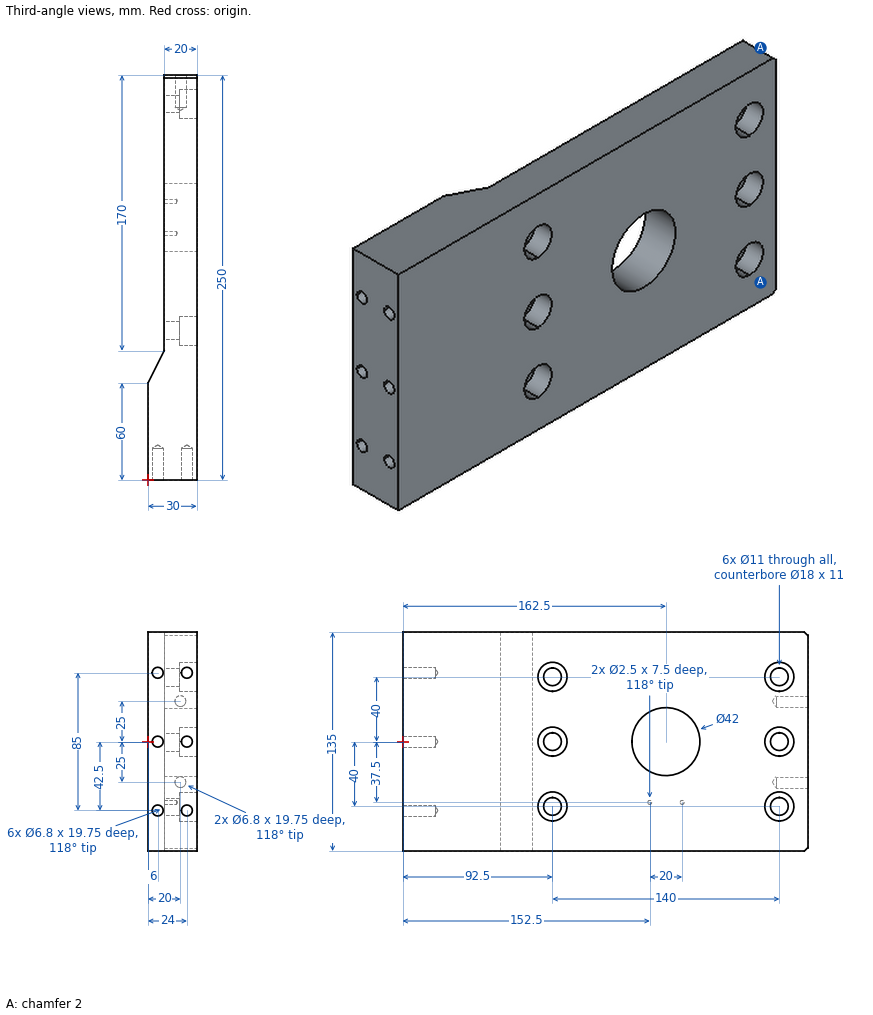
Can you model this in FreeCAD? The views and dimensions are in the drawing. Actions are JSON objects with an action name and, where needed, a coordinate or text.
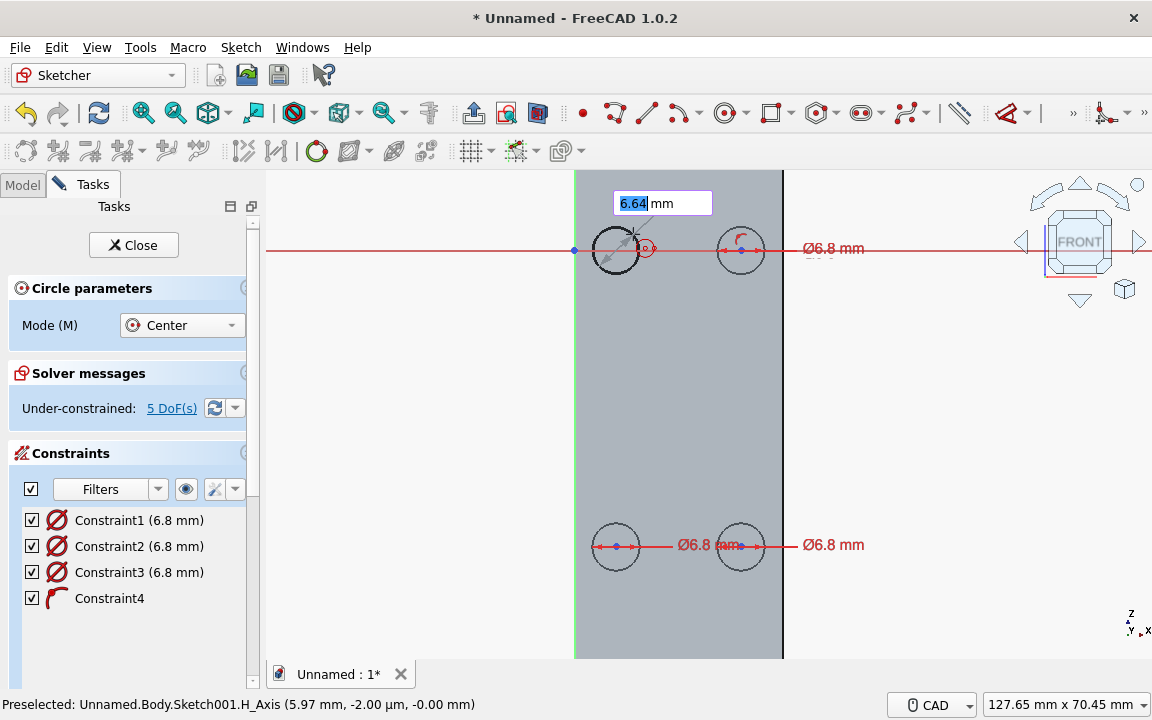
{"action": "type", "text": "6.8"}
{"action": "key", "text": "Return"}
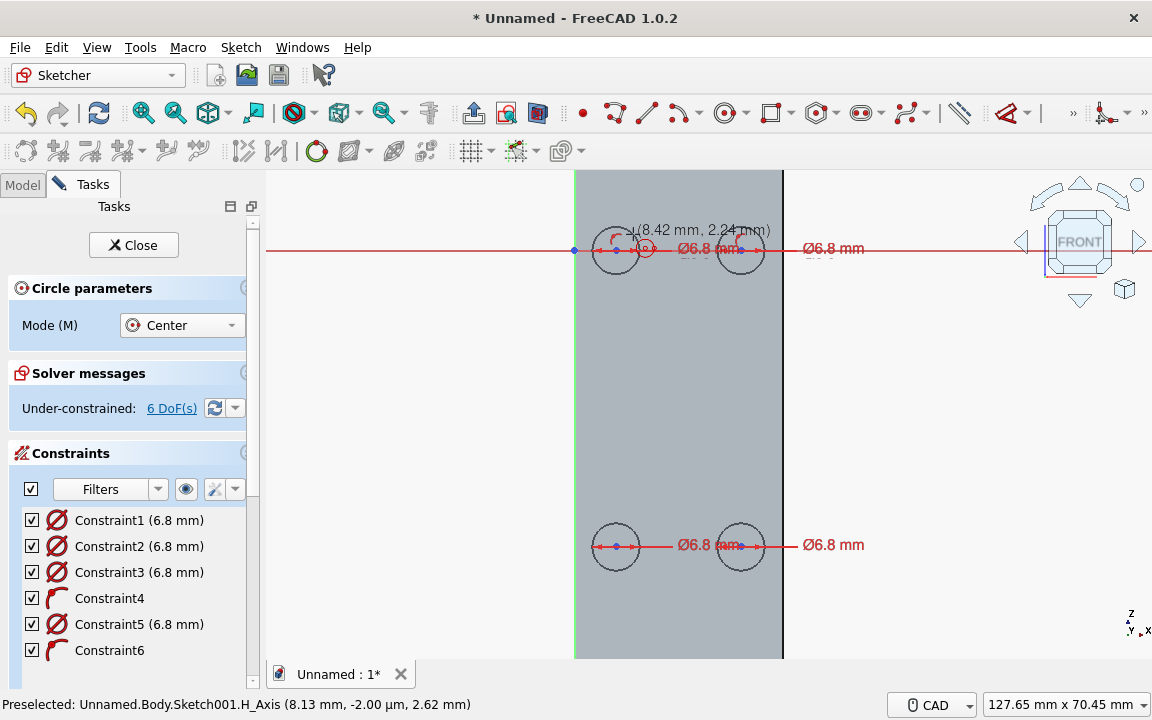
{"action": "scroll", "coordinate": [617, 548], "scroll_direction": "down", "scroll_amount": 4}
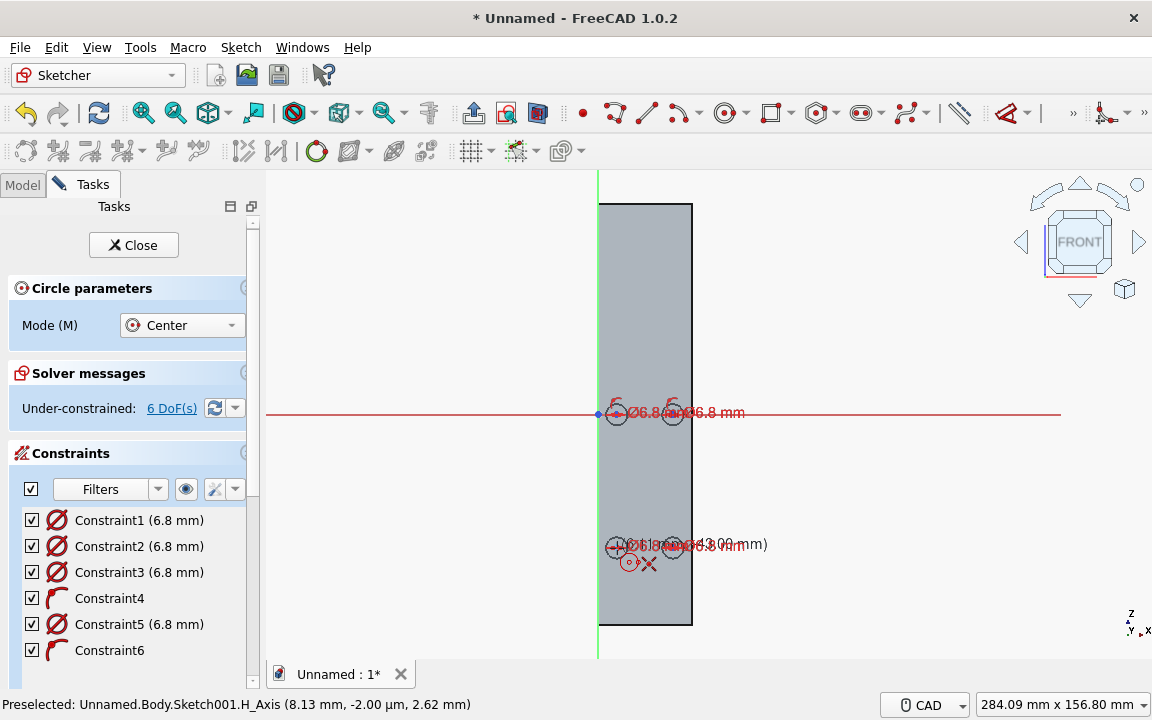
{"action": "scroll", "coordinate": [617, 282], "scroll_direction": "up", "scroll_amount": 4}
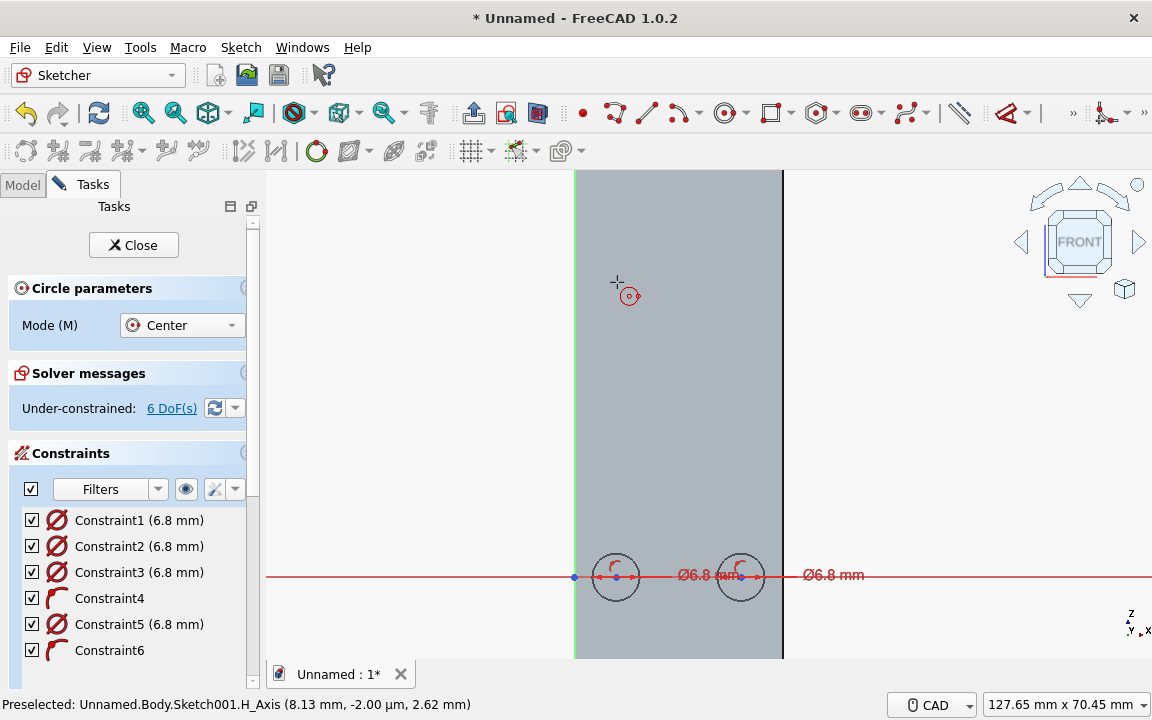
{"action": "left_click", "coordinate": [616, 282]}
{"action": "mouse_move", "coordinate": [633, 266]}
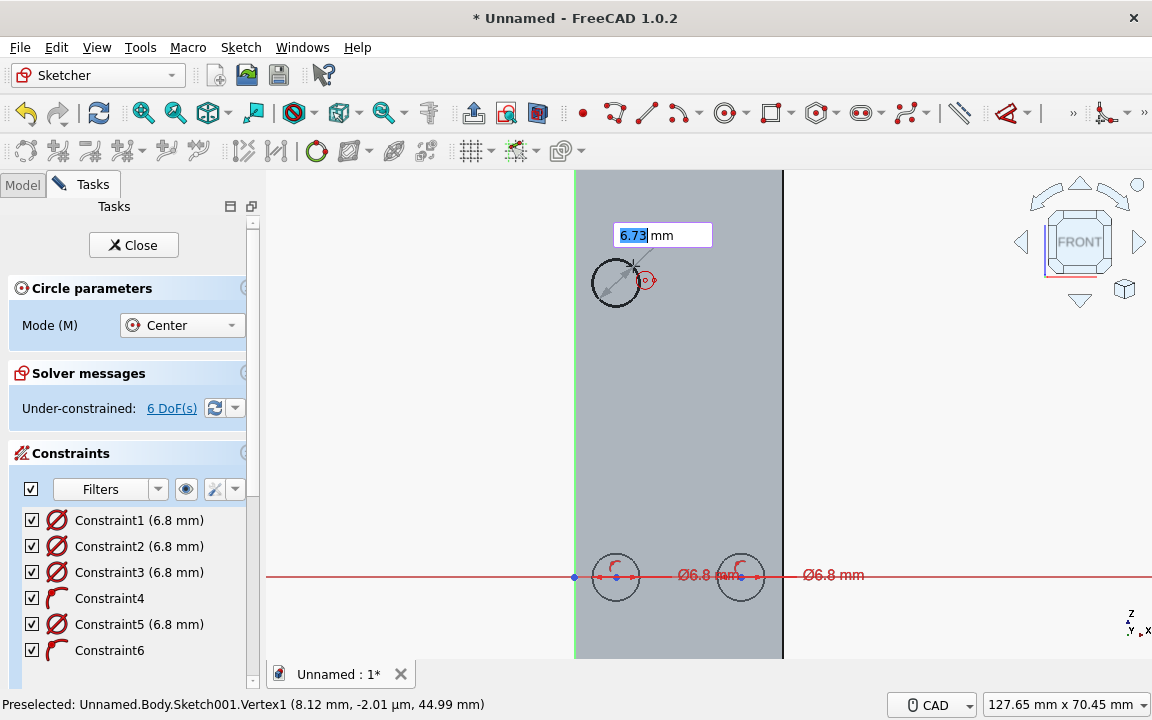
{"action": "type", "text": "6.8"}
{"action": "key", "text": "Return"}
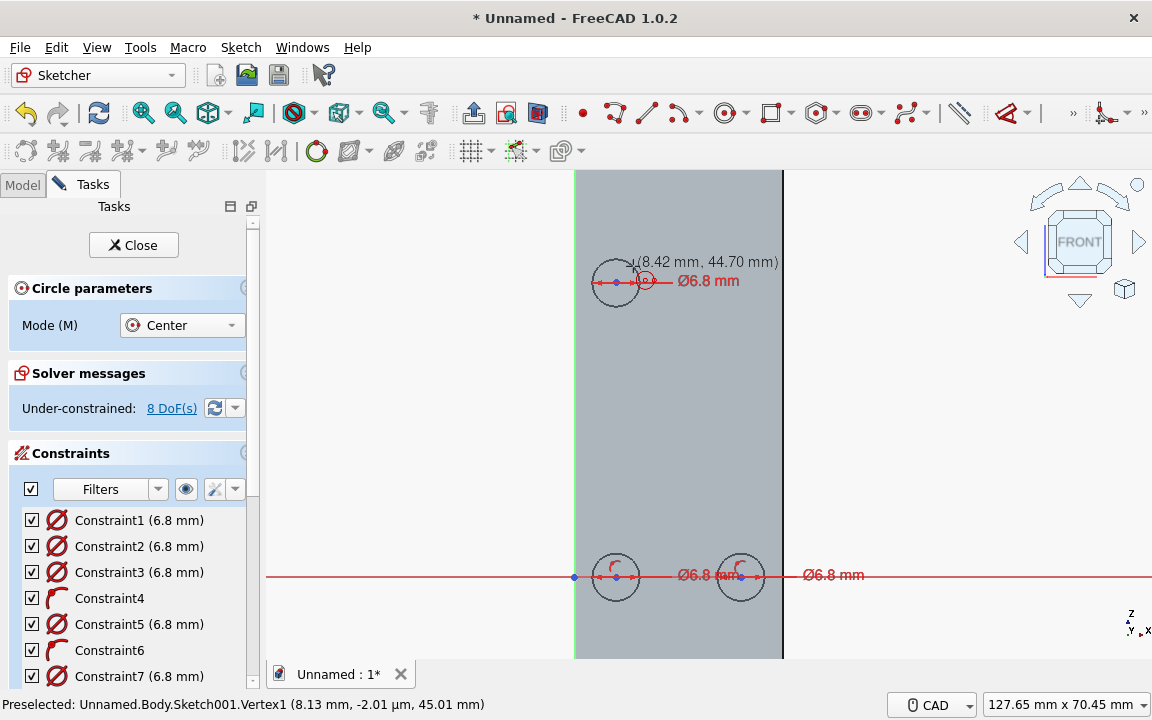
{"action": "left_click", "coordinate": [741, 282]}
{"action": "mouse_move", "coordinate": [758, 266]}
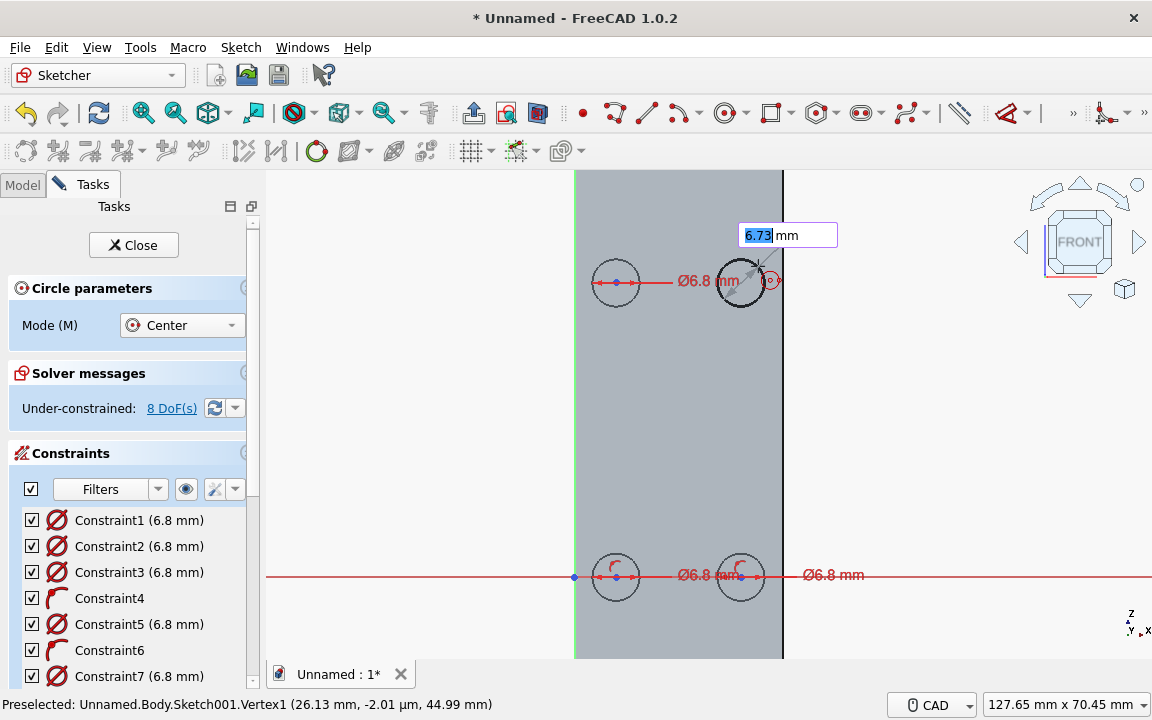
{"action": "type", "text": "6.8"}
{"action": "key", "text": "Return"}
{"action": "key", "text": "Escape"}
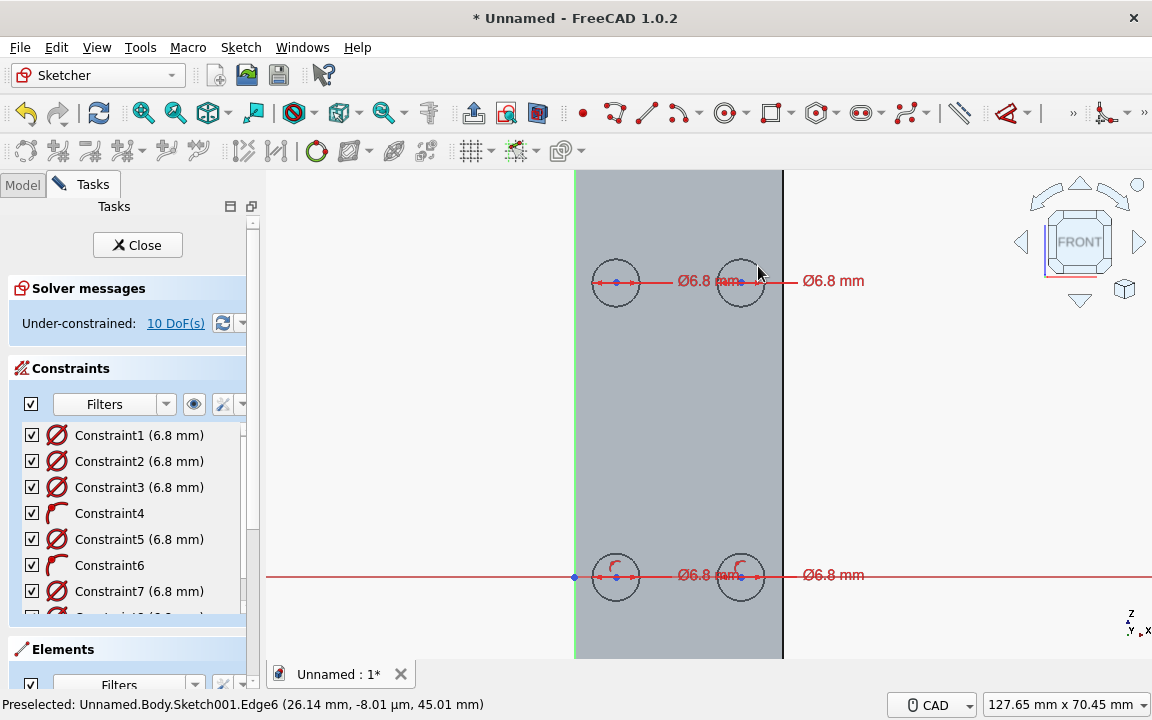
{"action": "scroll", "coordinate": [617, 282], "scroll_direction": "down", "scroll_amount": 4}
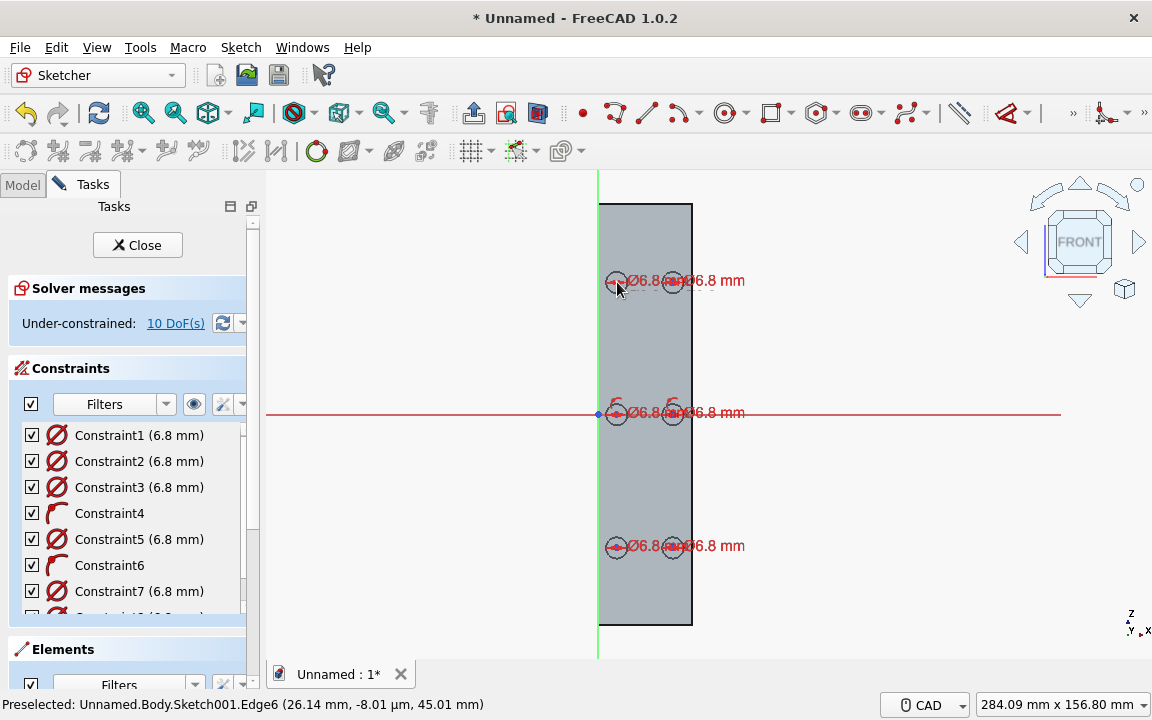
{"action": "left_click", "coordinate": [617, 548]}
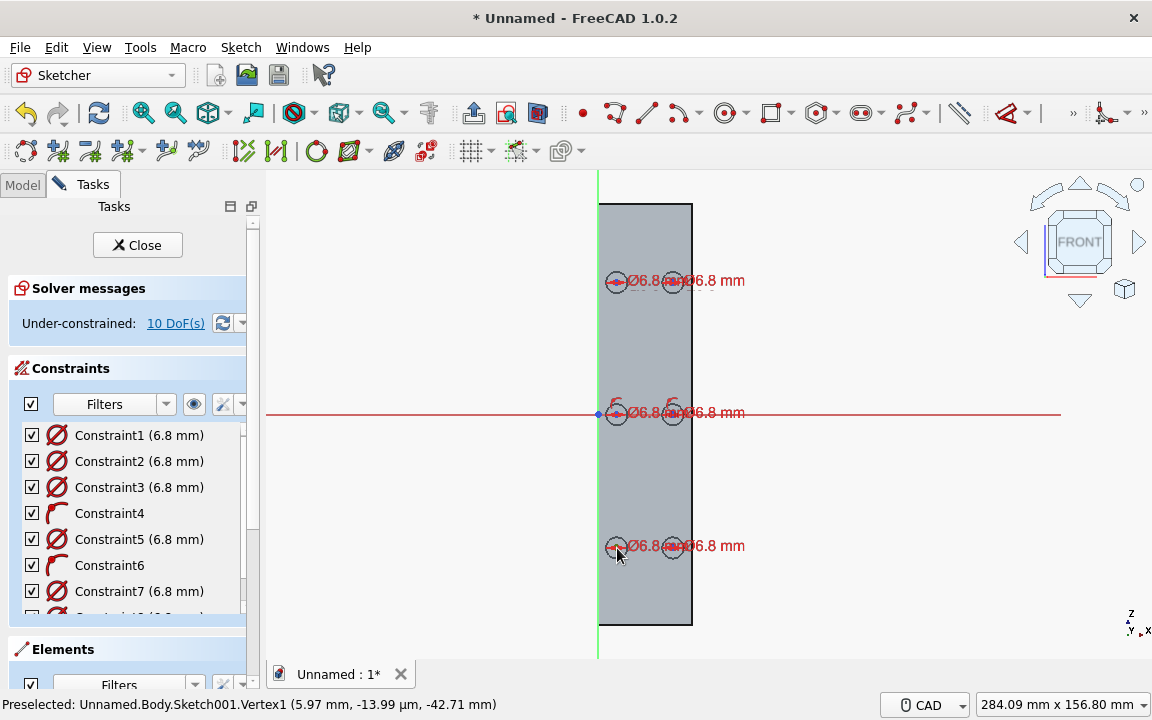
{"action": "left_click", "coordinate": [673, 548]}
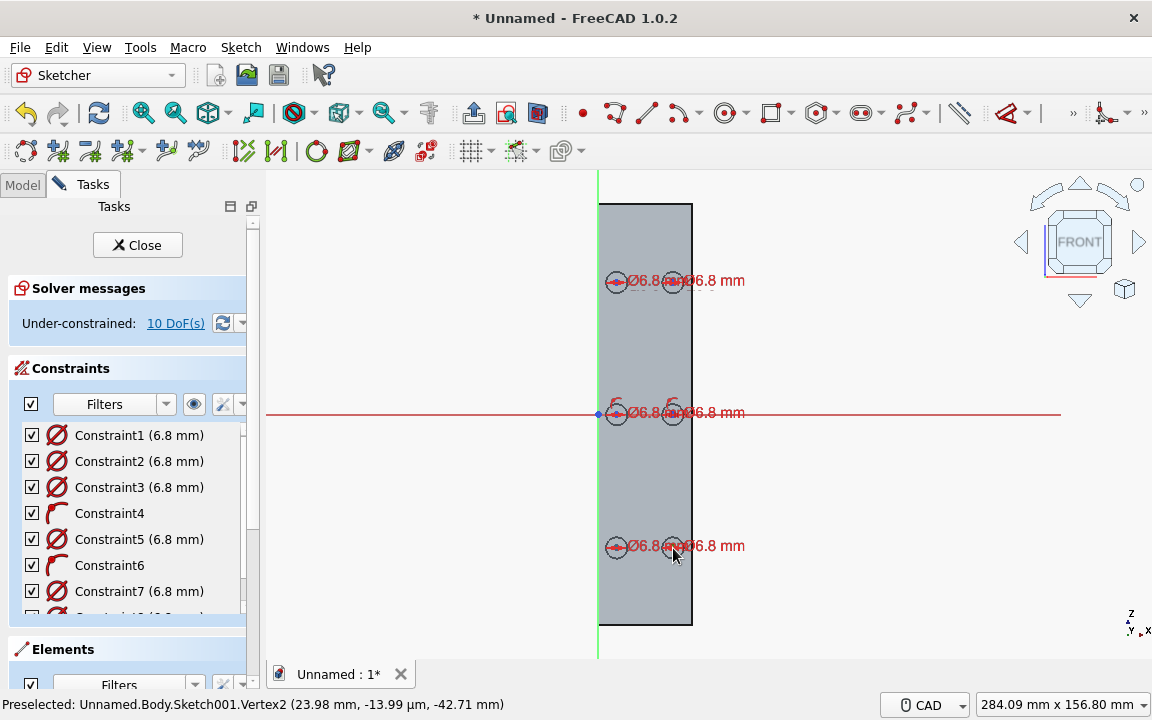
{"action": "key", "text": "h"}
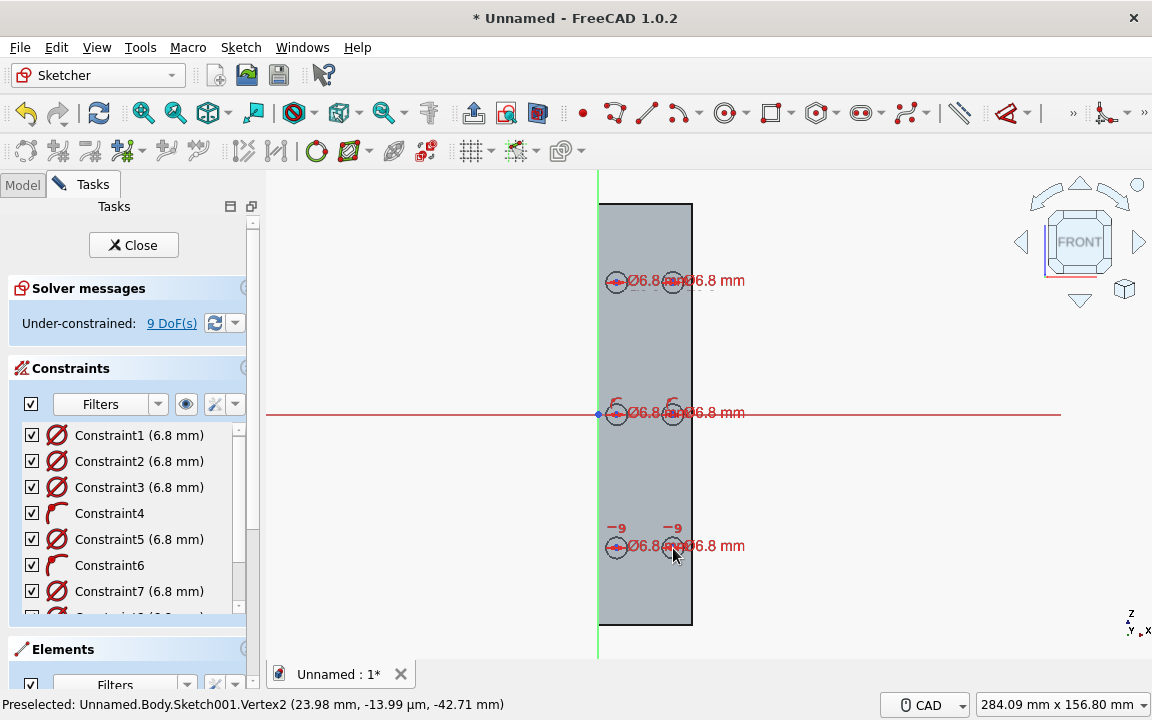
{"action": "left_click", "coordinate": [673, 548]}